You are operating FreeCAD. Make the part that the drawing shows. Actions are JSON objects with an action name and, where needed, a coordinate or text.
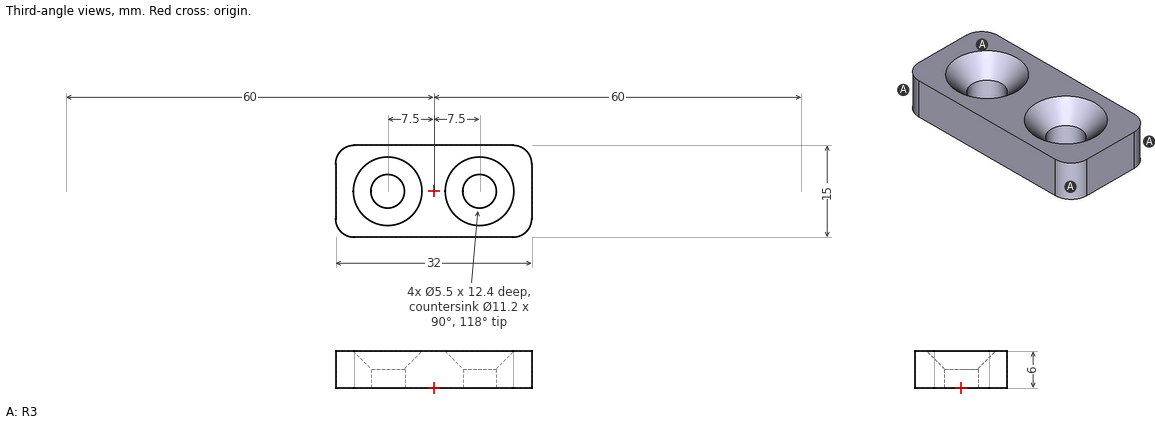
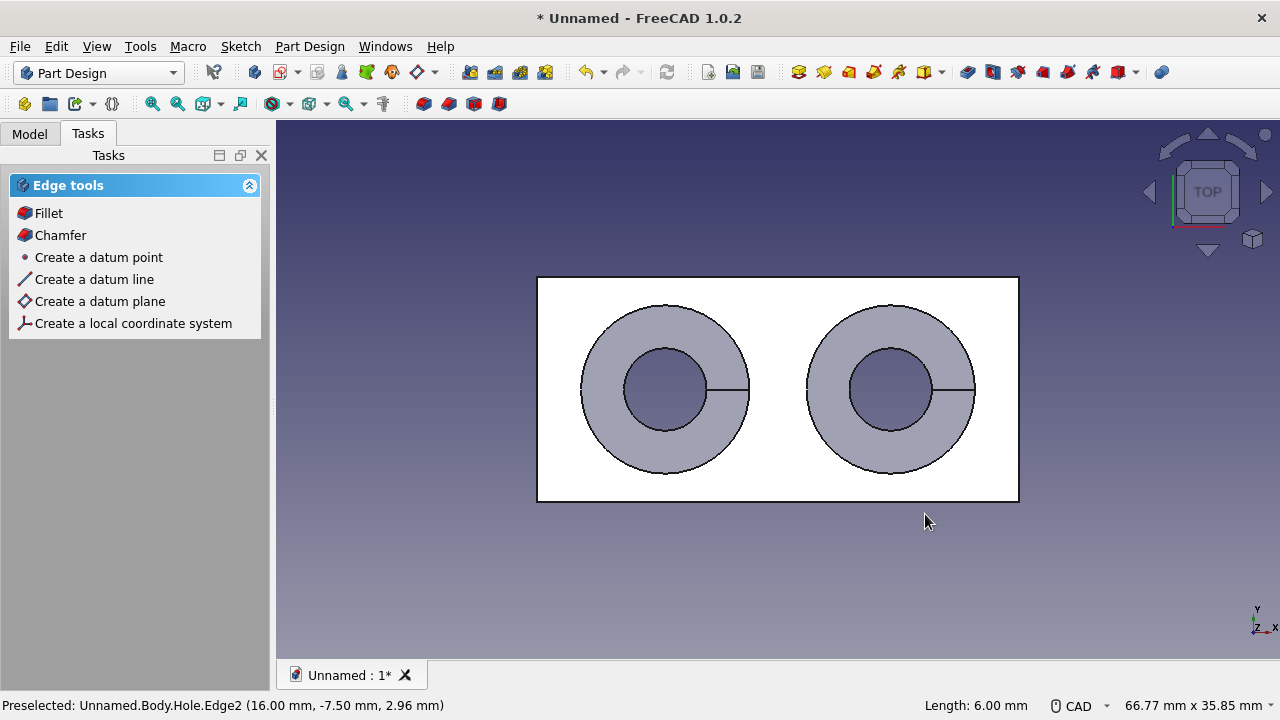
{"action": "key", "text": "1"}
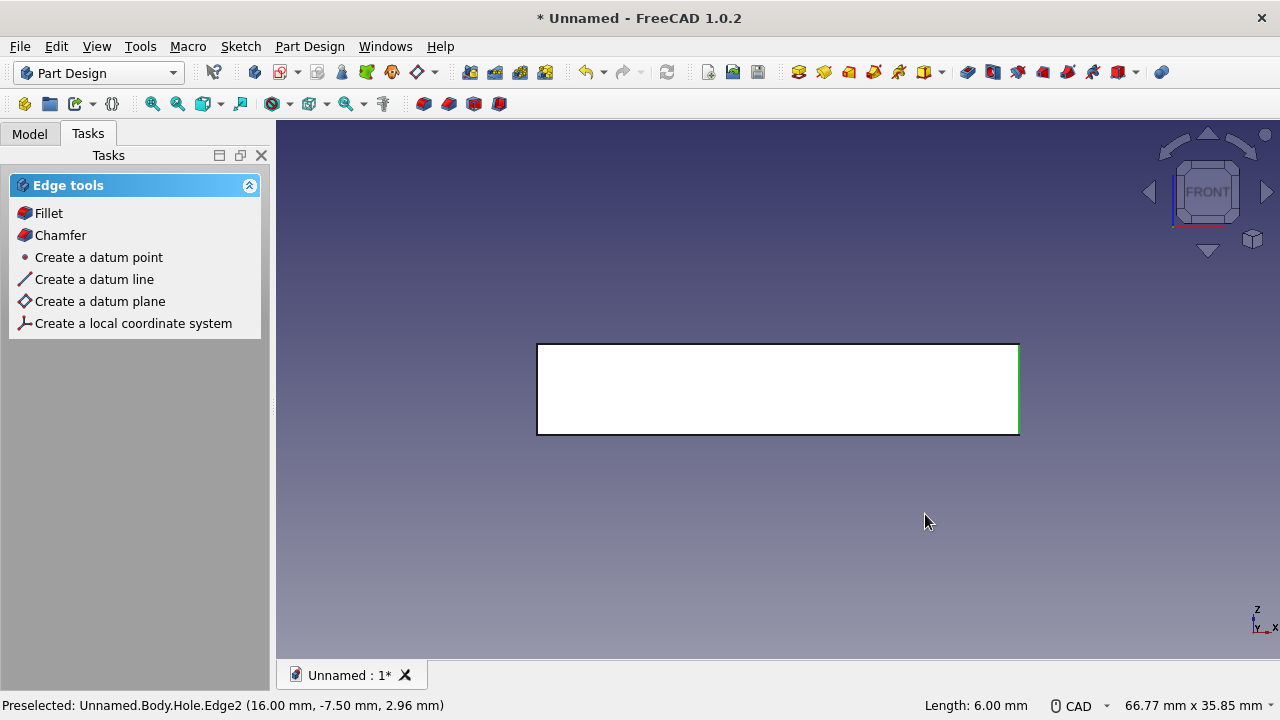
{"action": "left_click", "coordinate": [537, 388], "text": "ctrl"}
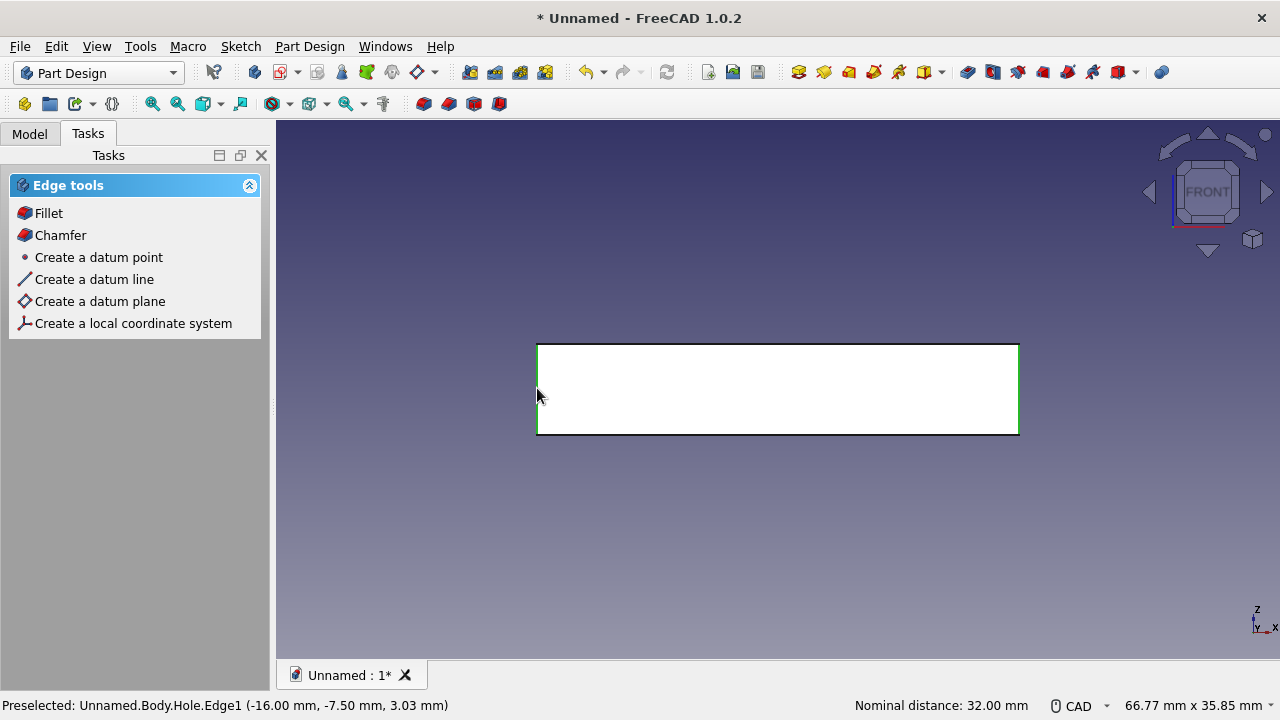
{"action": "key", "text": "3"}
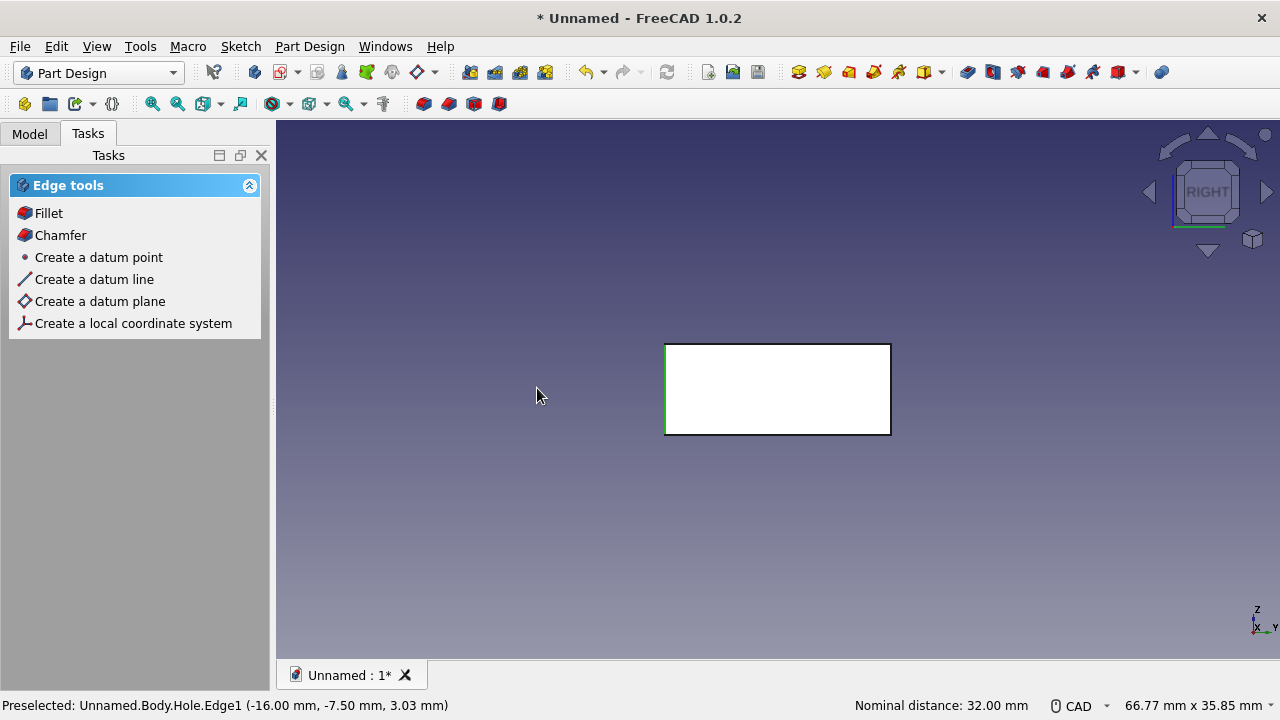
{"action": "left_click", "coordinate": [153, 104]}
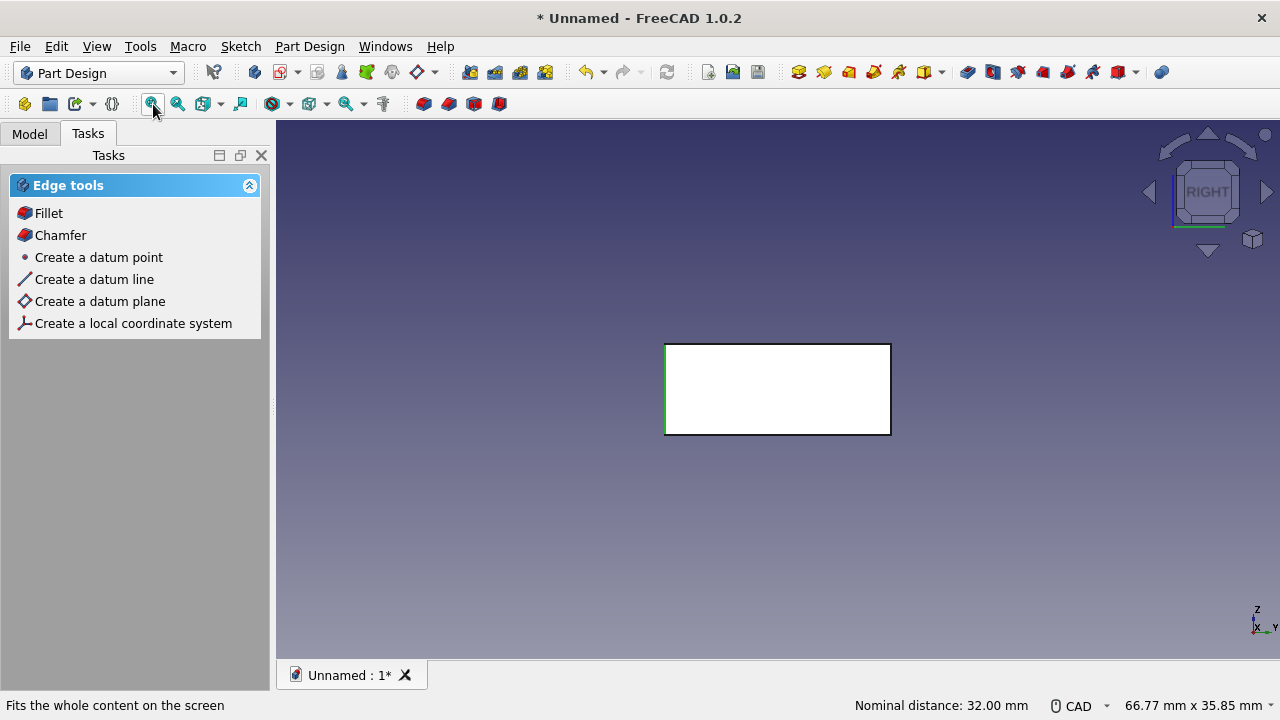
{"action": "left_click", "coordinate": [891, 388], "text": "ctrl"}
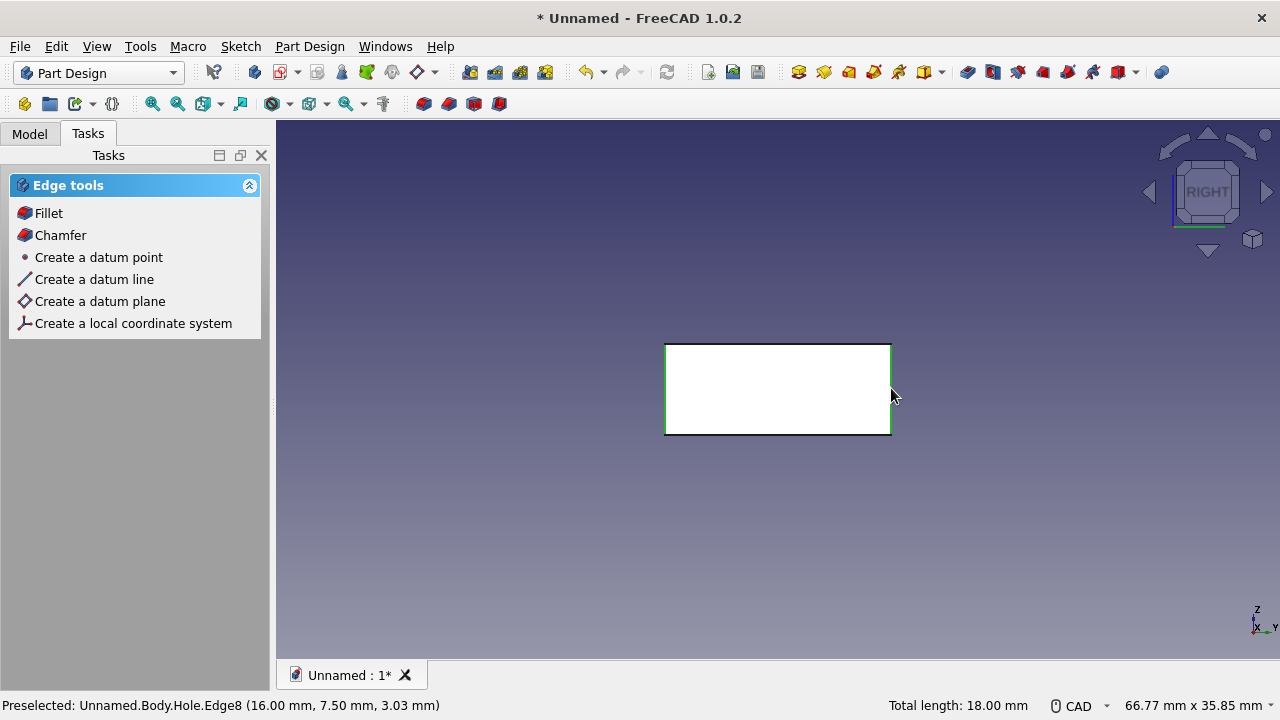
{"action": "key", "text": "5"}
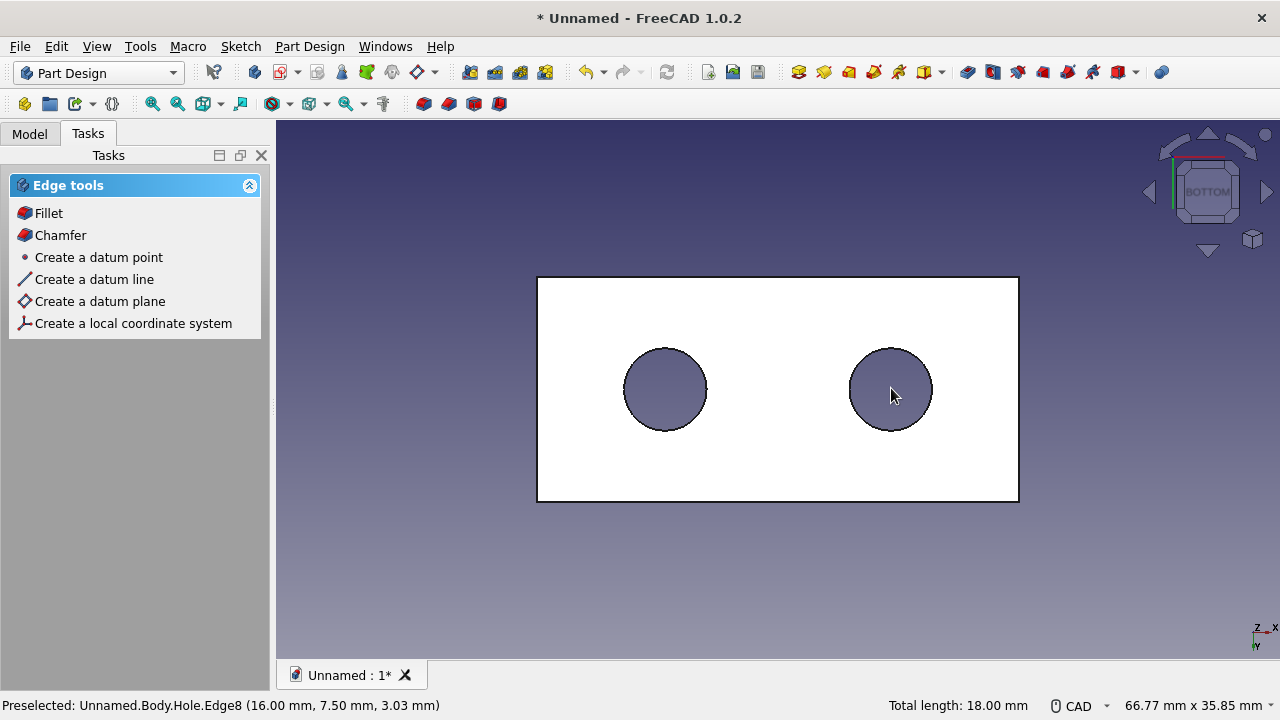
{"action": "key", "text": "4"}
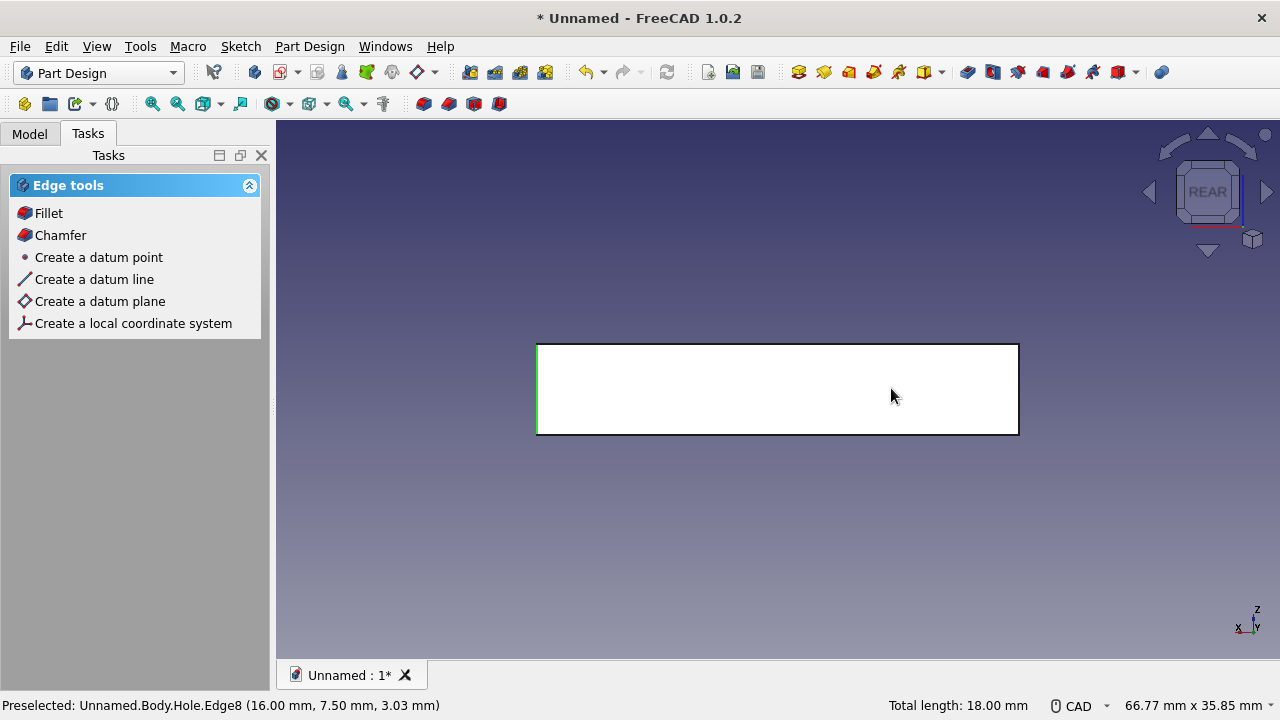
{"action": "left_click", "coordinate": [1019, 388], "text": "ctrl"}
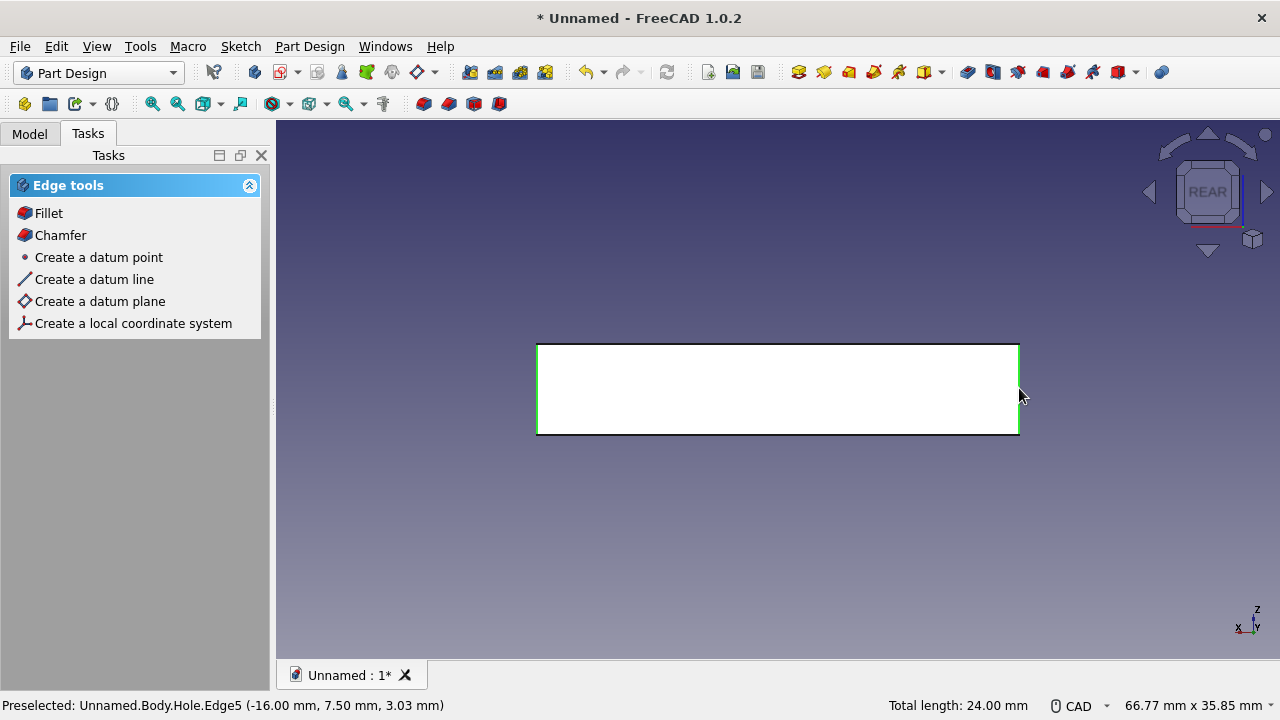
{"action": "left_click", "coordinate": [424, 104]}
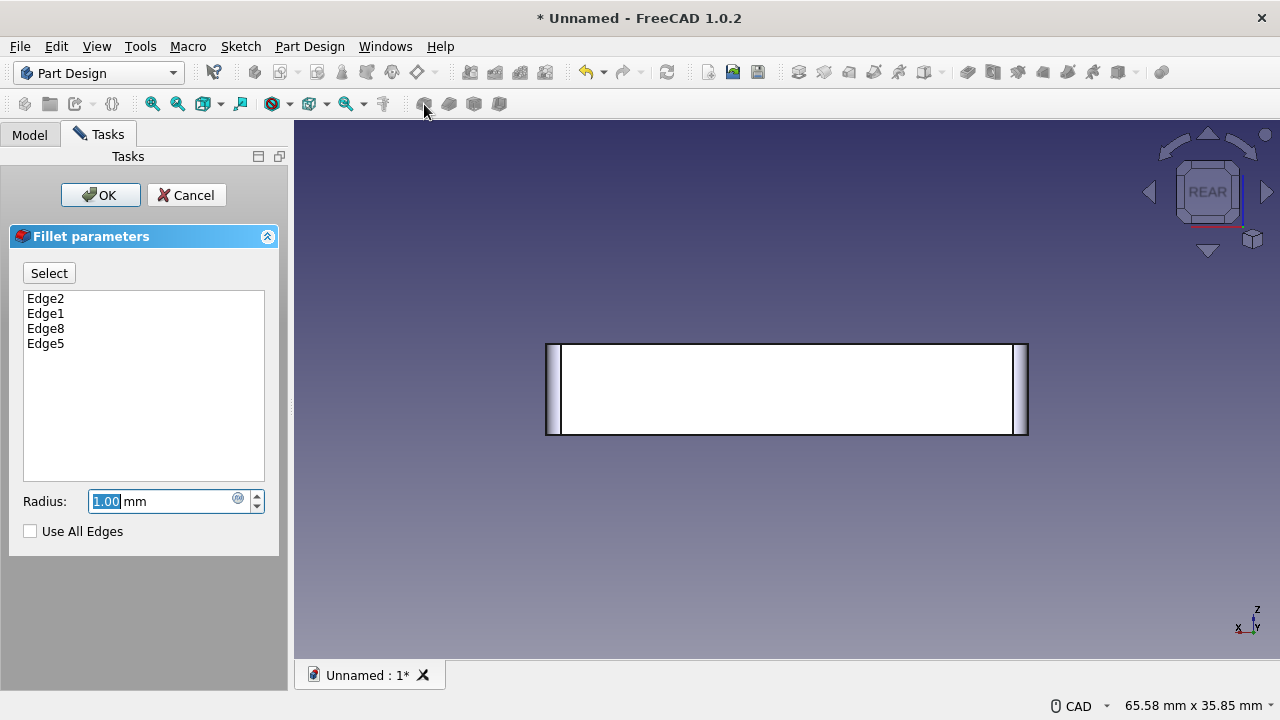
{"action": "type", "text": "3"}
{"action": "key", "text": "Tab"}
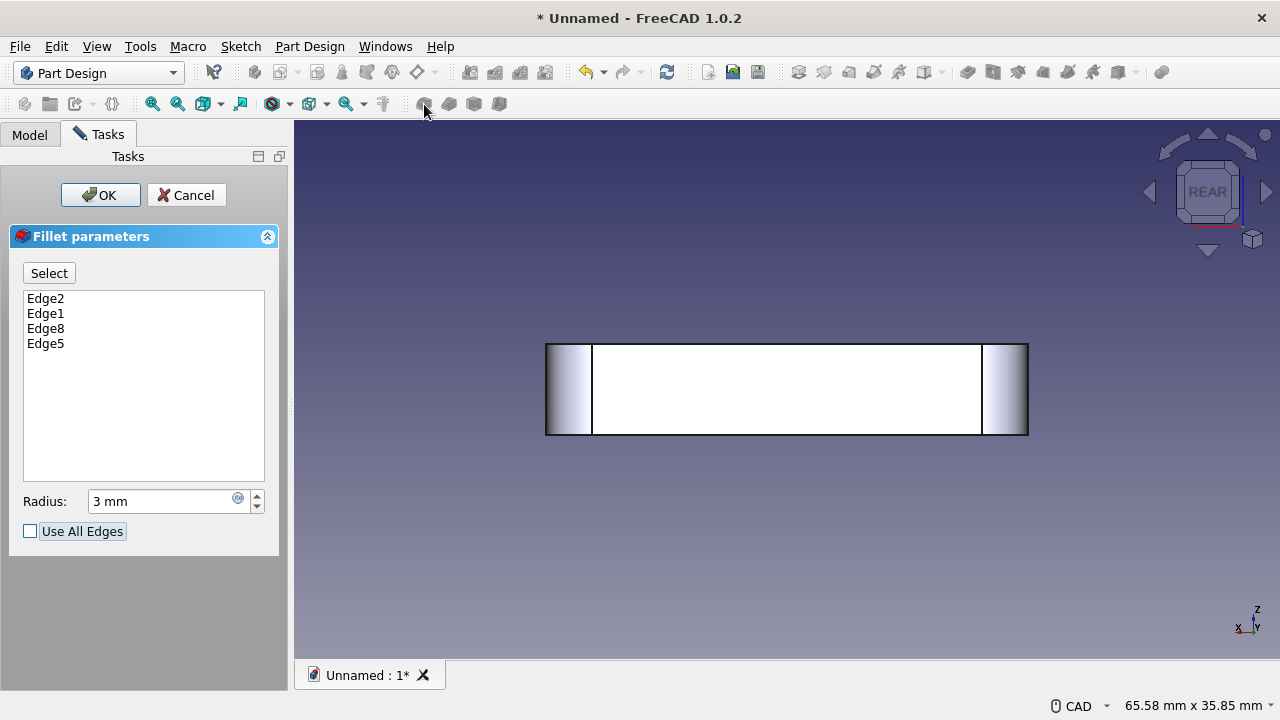
{"action": "left_click", "coordinate": [101, 195]}